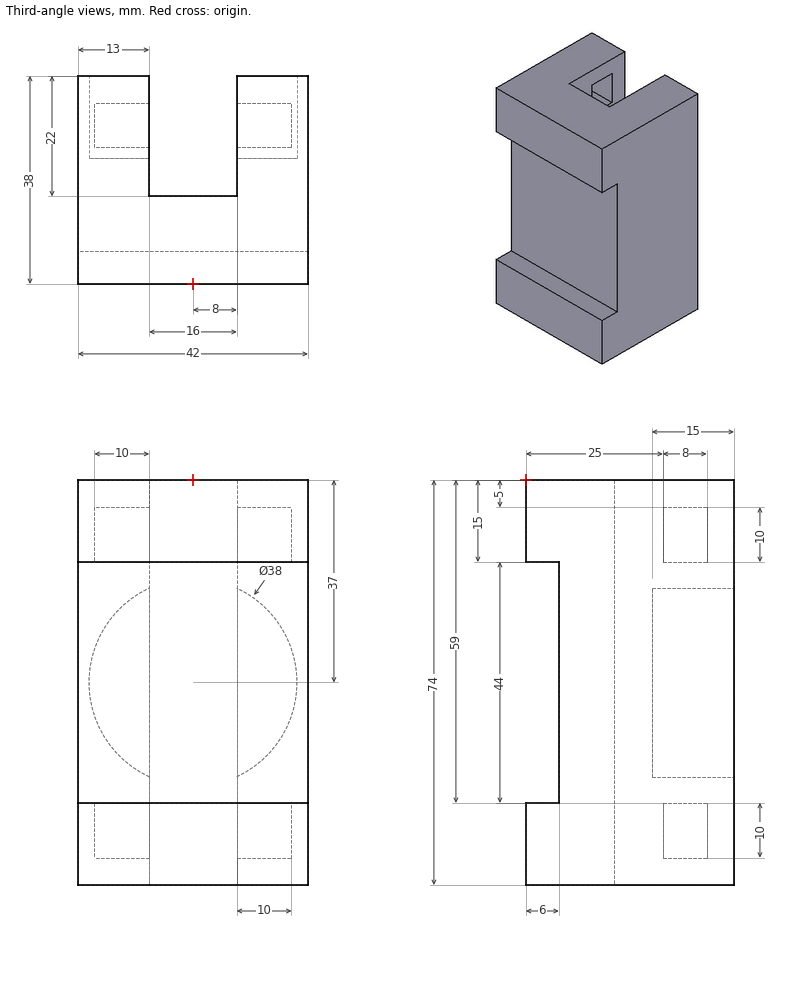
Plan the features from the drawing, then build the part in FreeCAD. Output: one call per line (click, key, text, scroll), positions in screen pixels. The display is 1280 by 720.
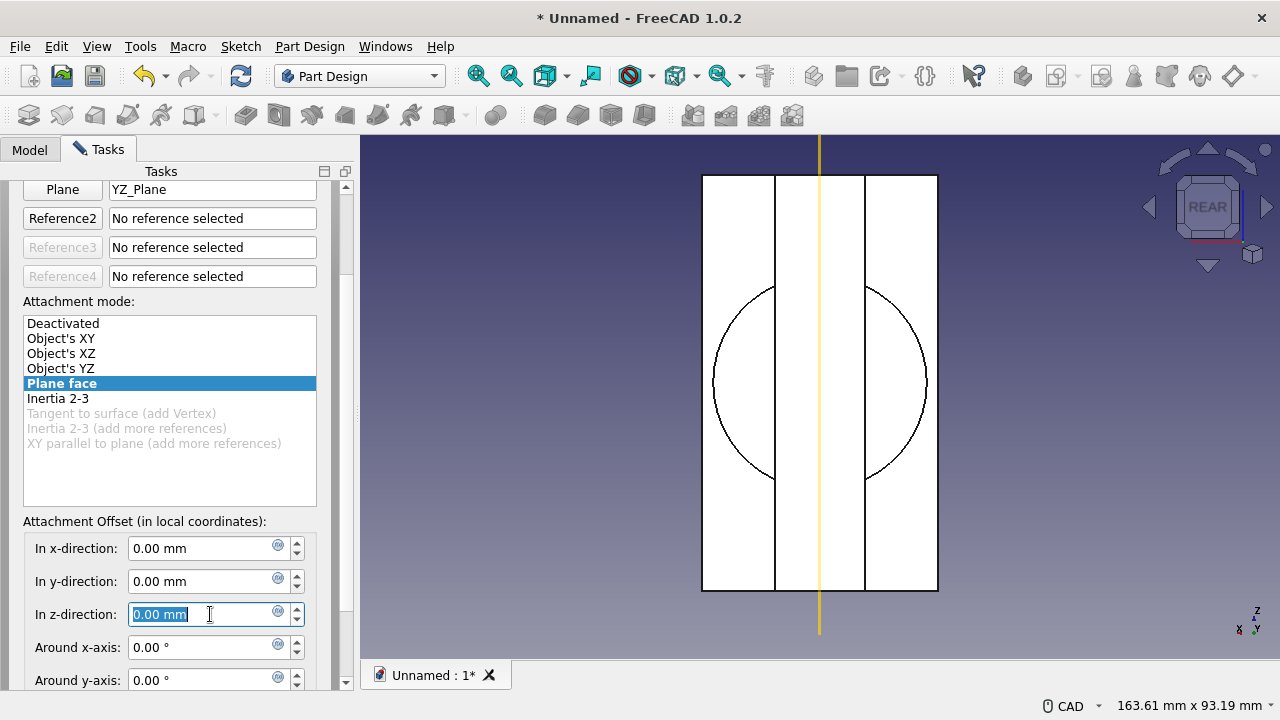
text(8)
key(Tab)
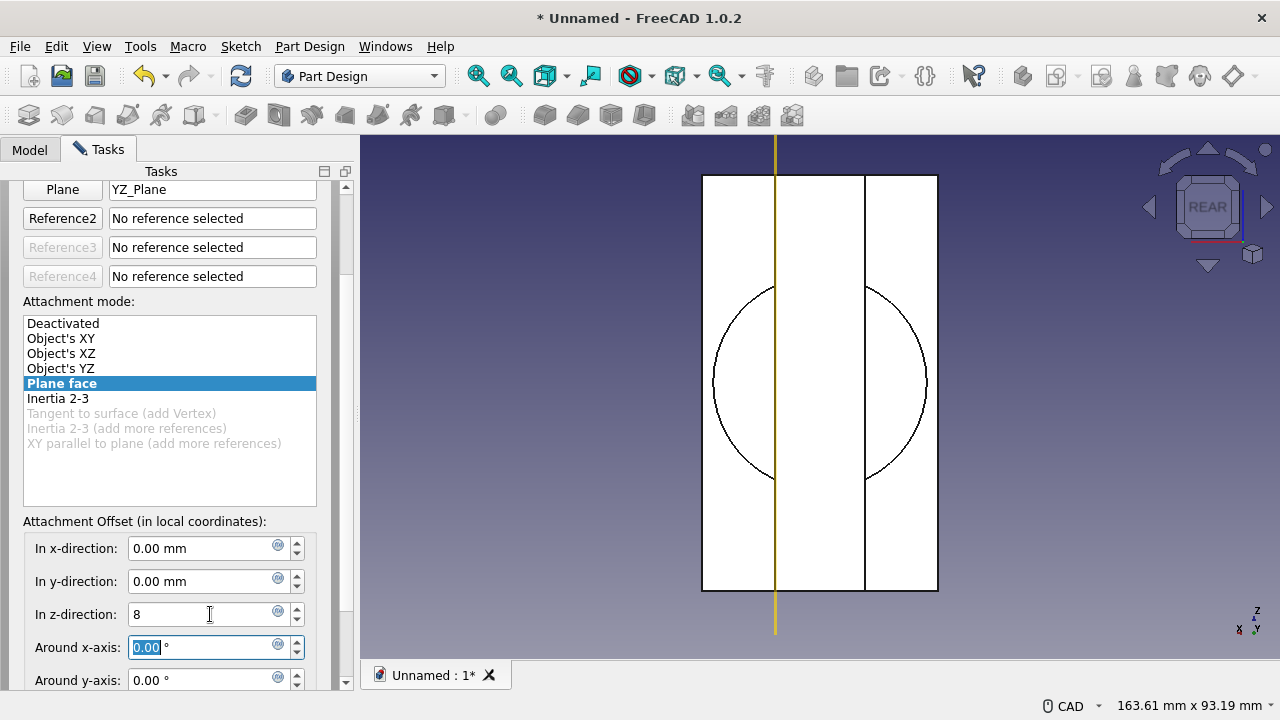
scroll(346, 436, up, 3)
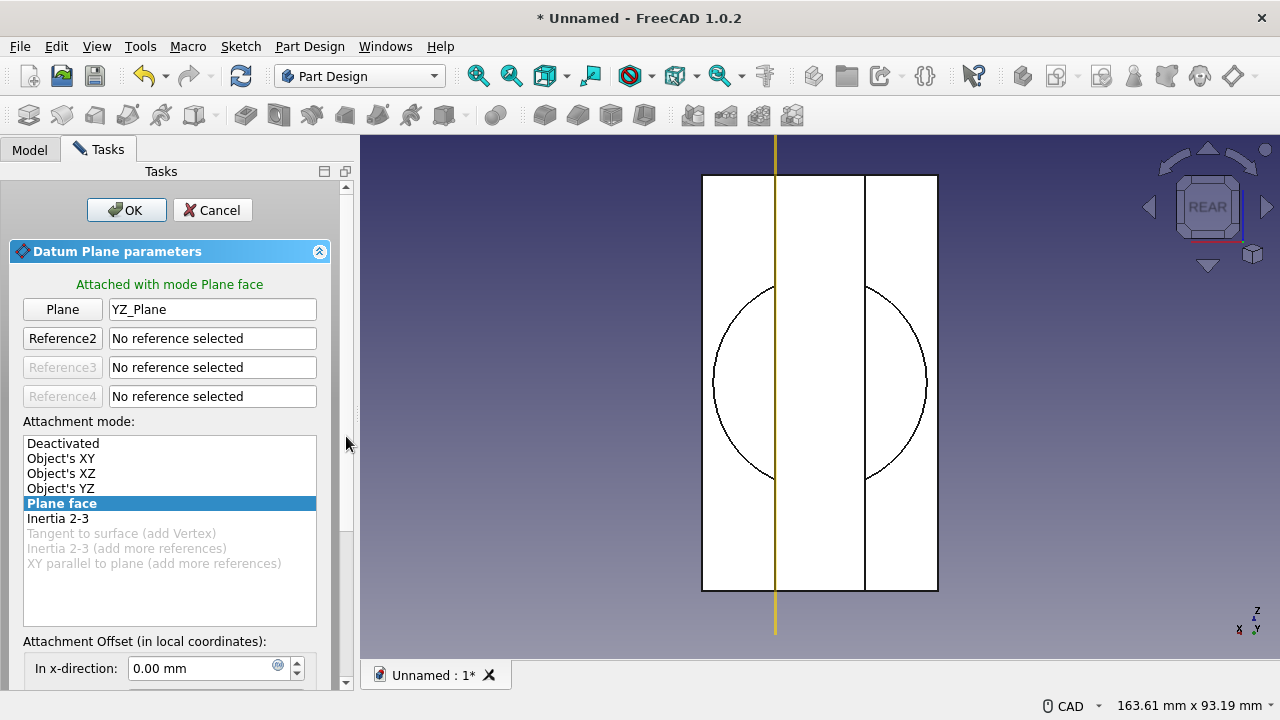
click(127, 210)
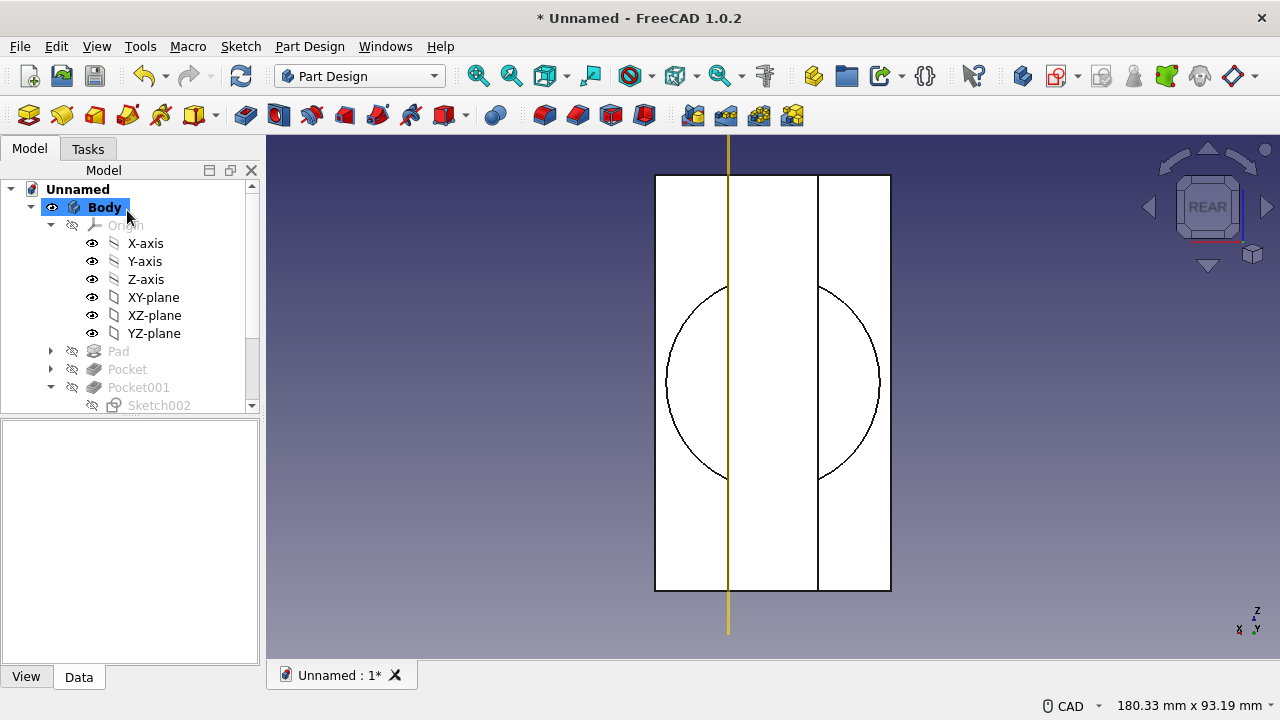
scroll(101, 293, down, 3)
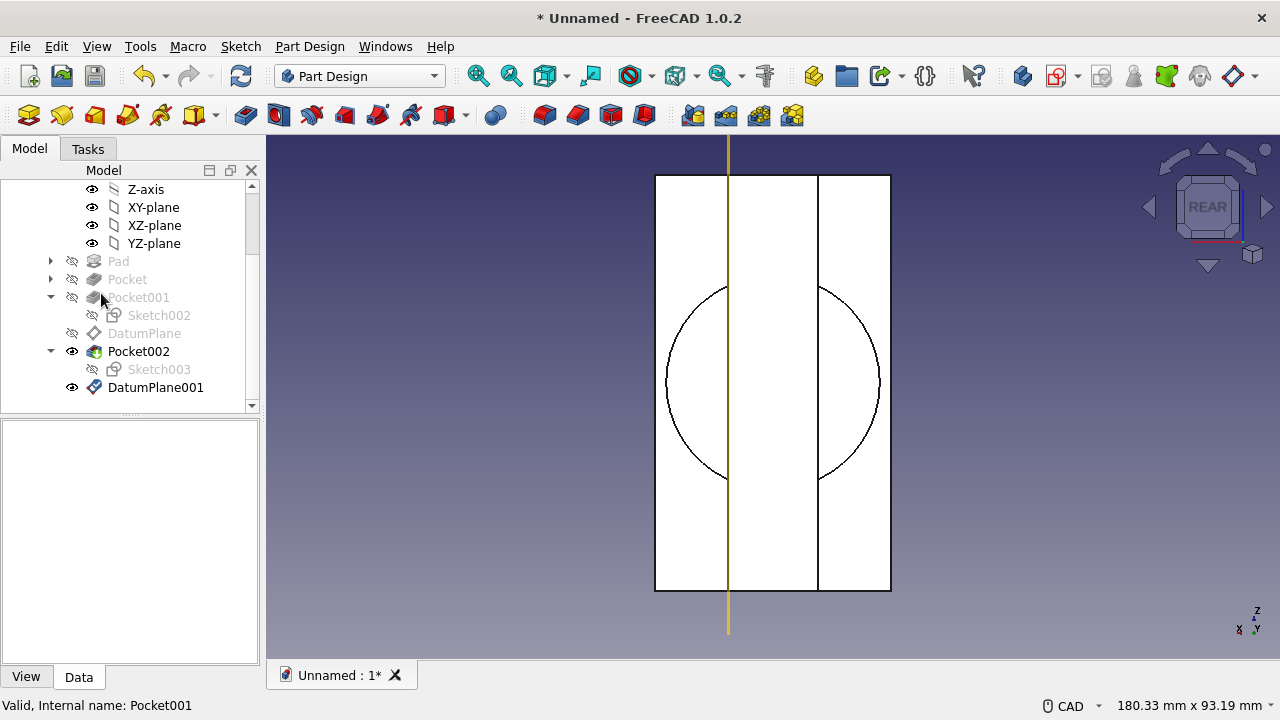
click(117, 387)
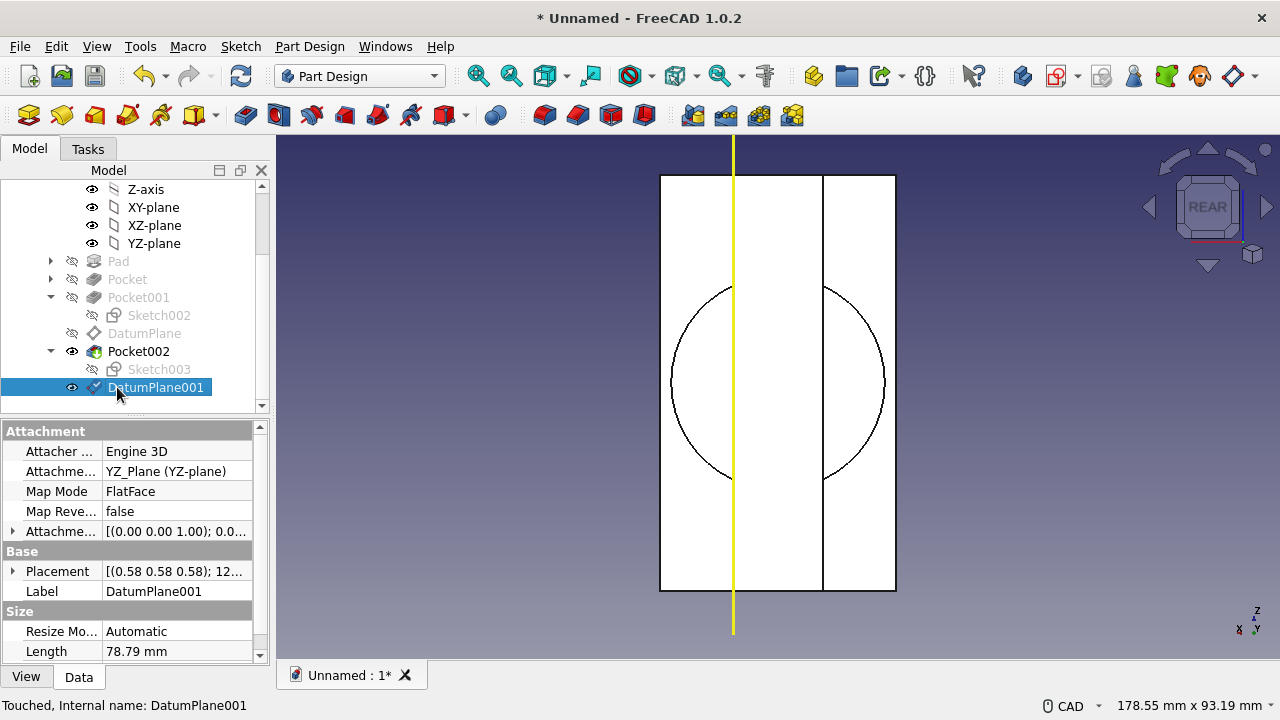
click(1056, 76)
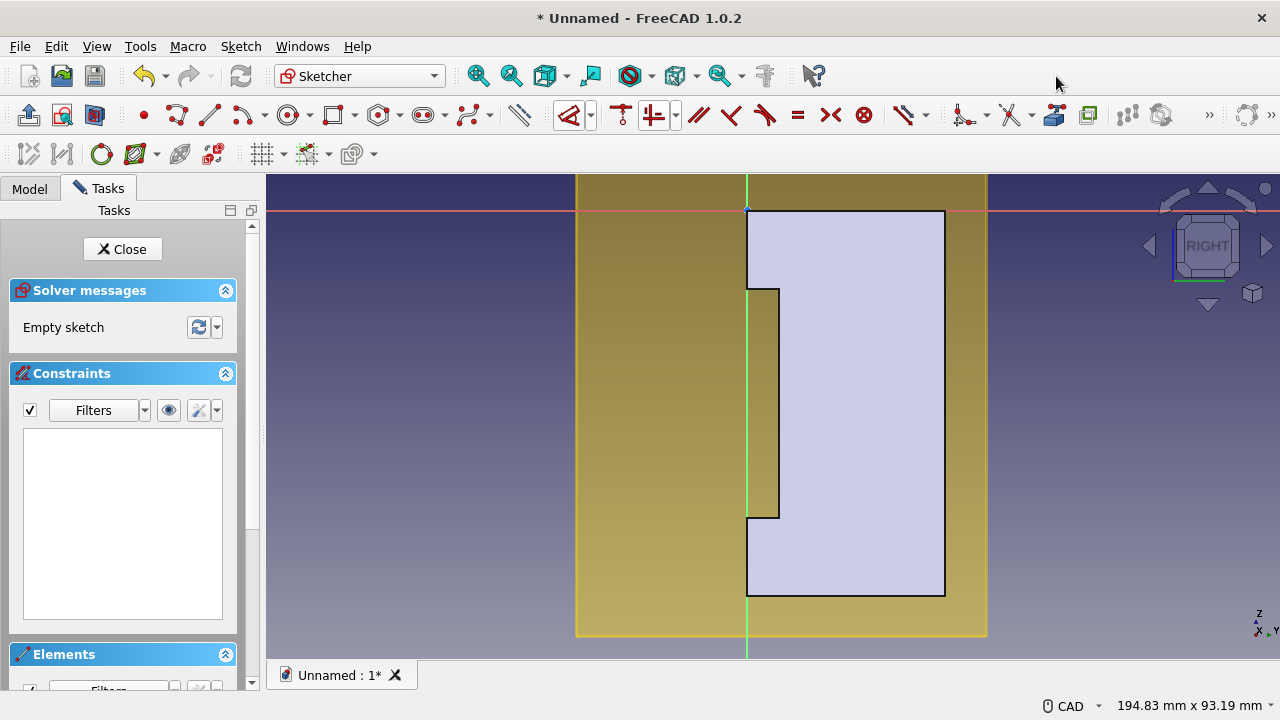
key(q)
key(s)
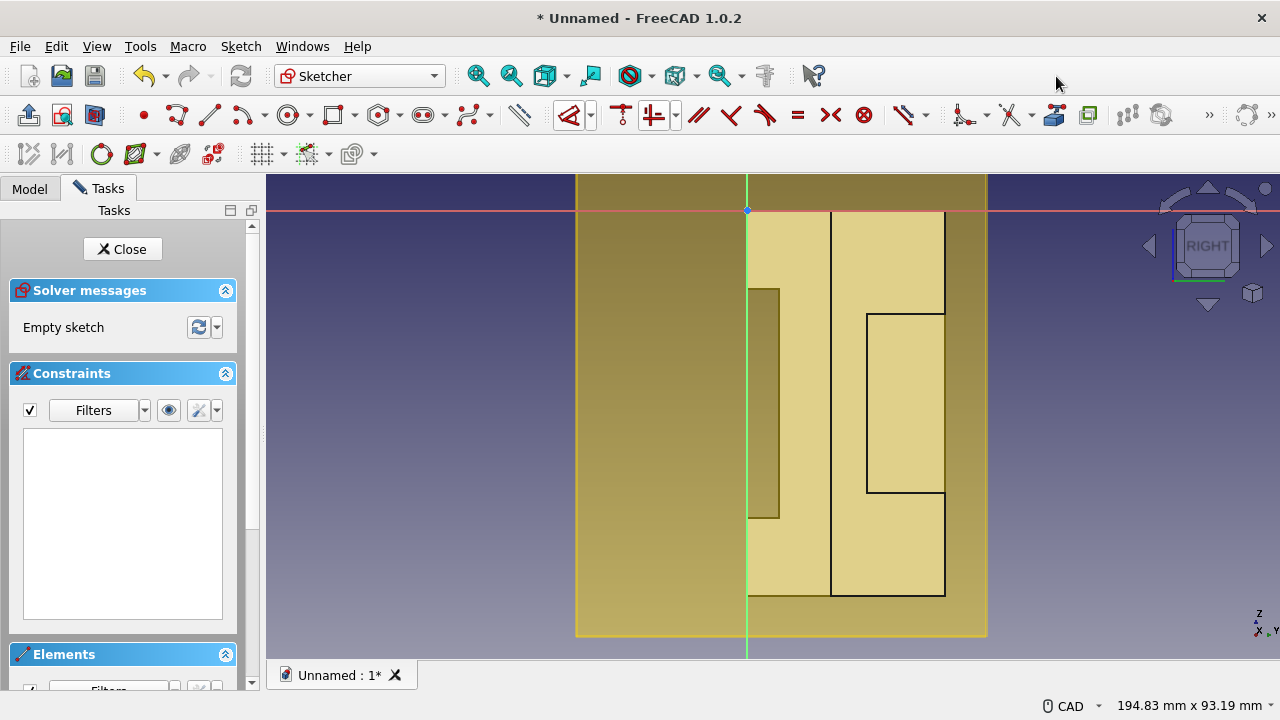
scroll(294, 535, down, 1)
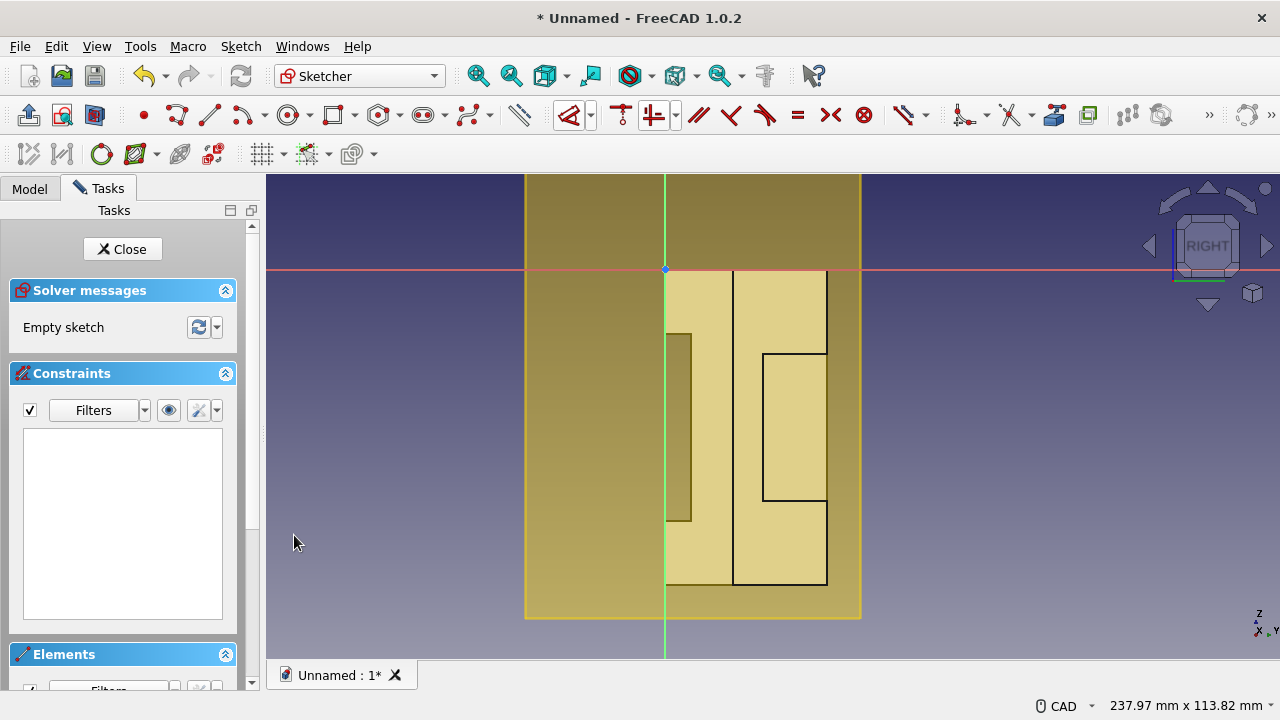
key(g)
key(r)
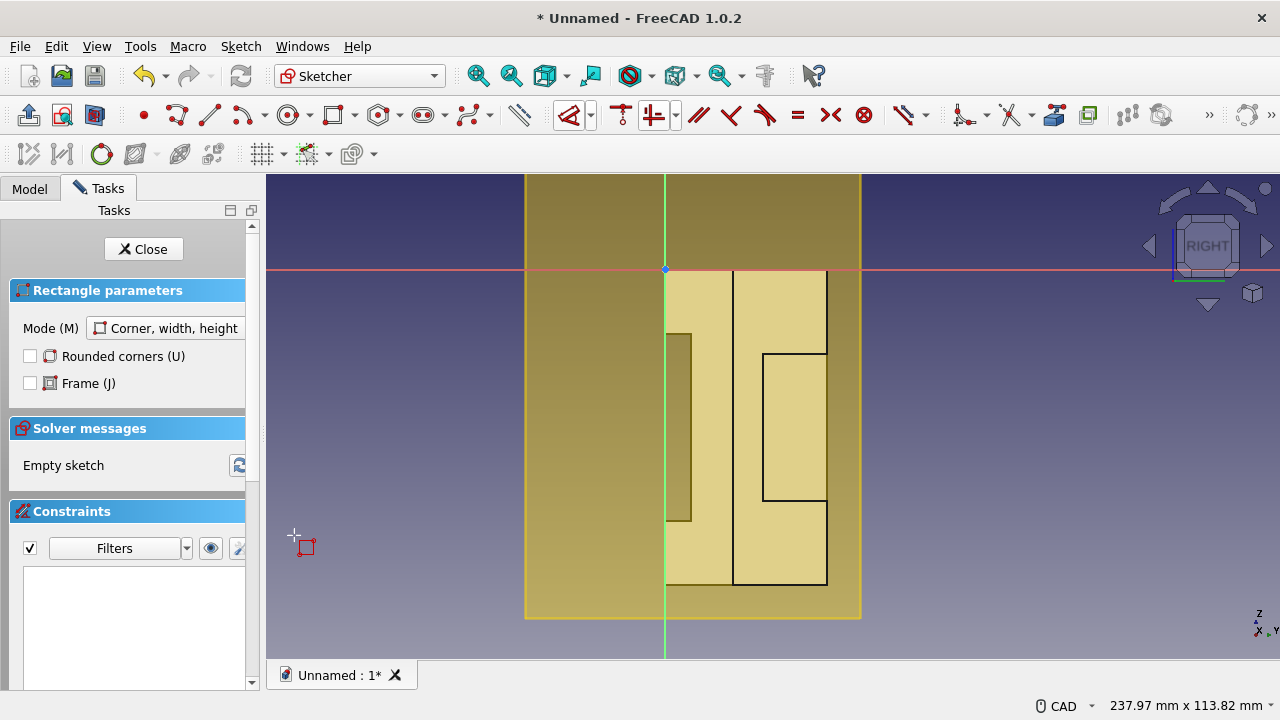
click(772, 521)
move(806, 564)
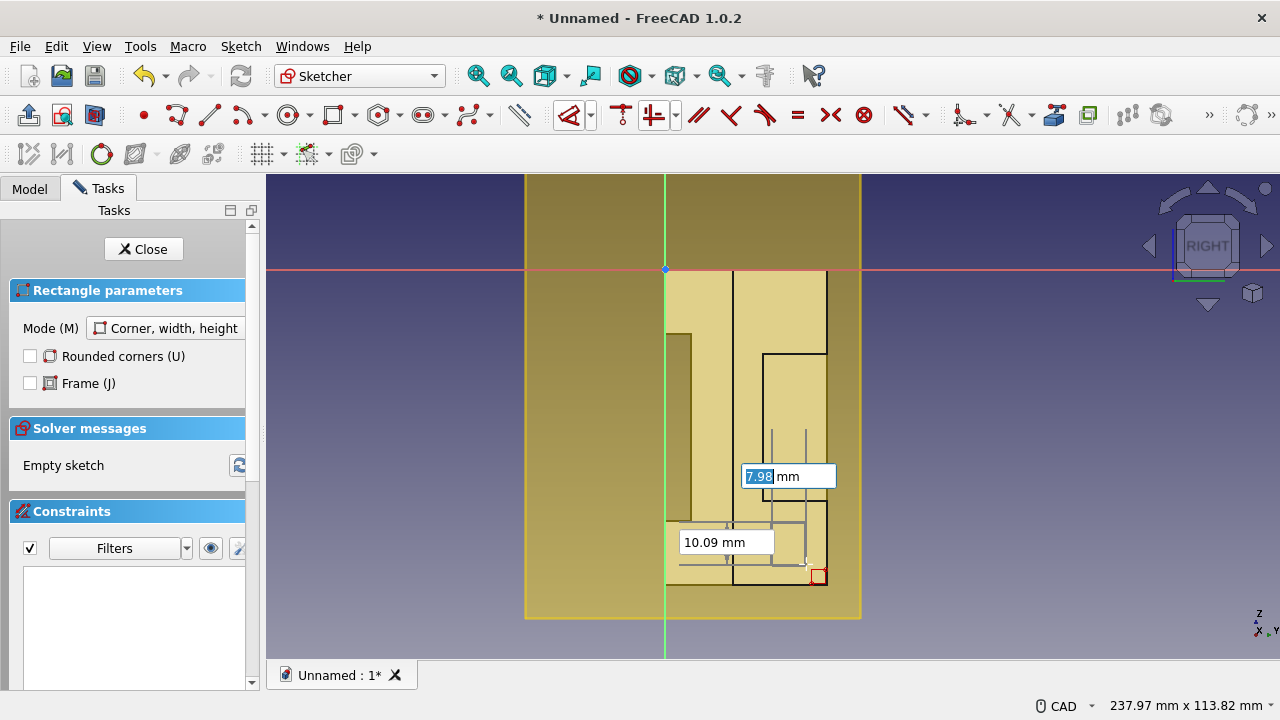
text(8)
key(Tab)
text(10)
key(Return)